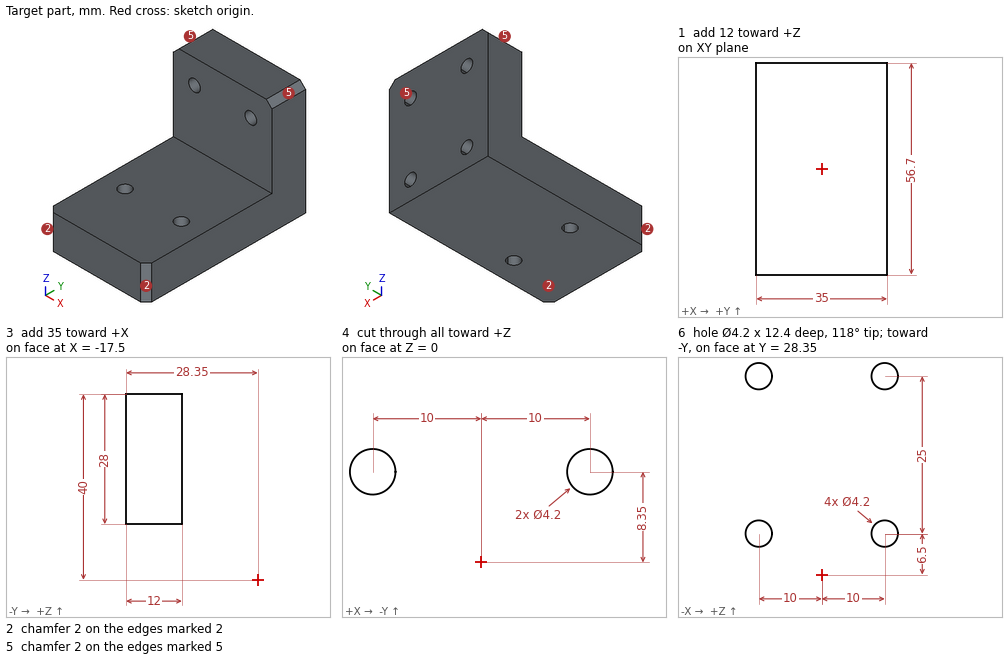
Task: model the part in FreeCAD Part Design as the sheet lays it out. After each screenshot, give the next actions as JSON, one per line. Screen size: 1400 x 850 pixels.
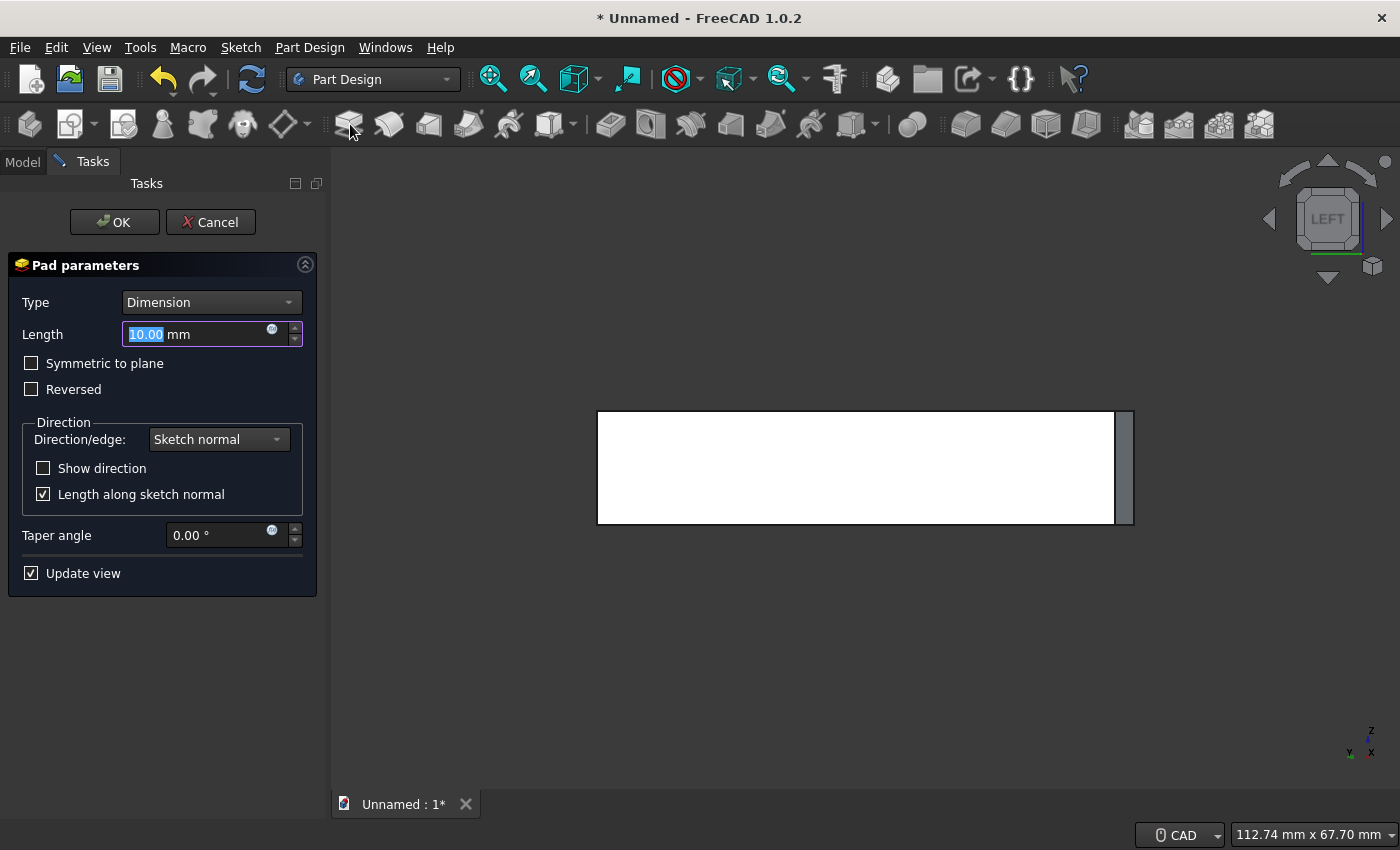
{"action": "type", "text": "35"}
{"action": "key", "text": "Tab"}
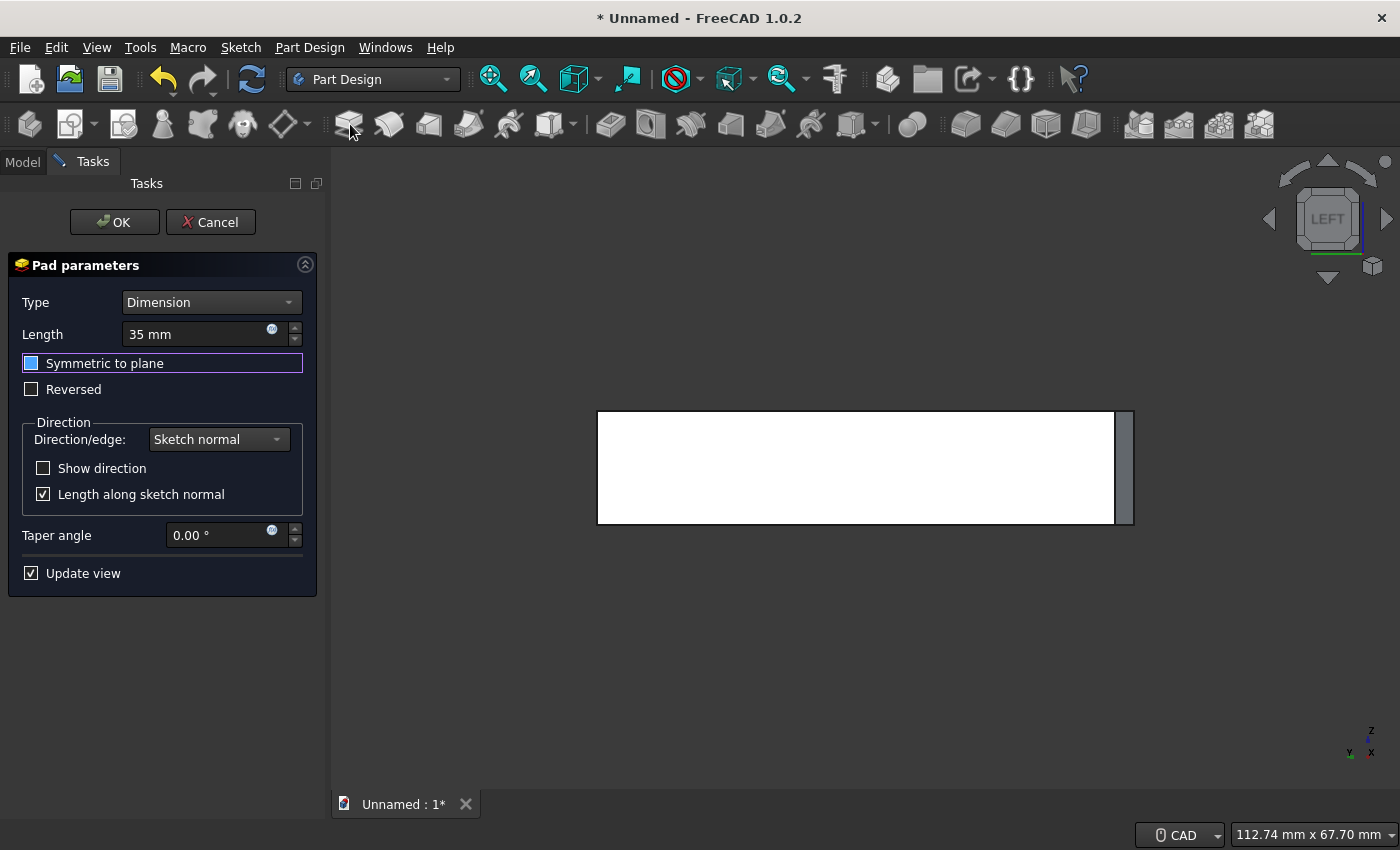
{"action": "left_click", "coordinate": [30, 389]}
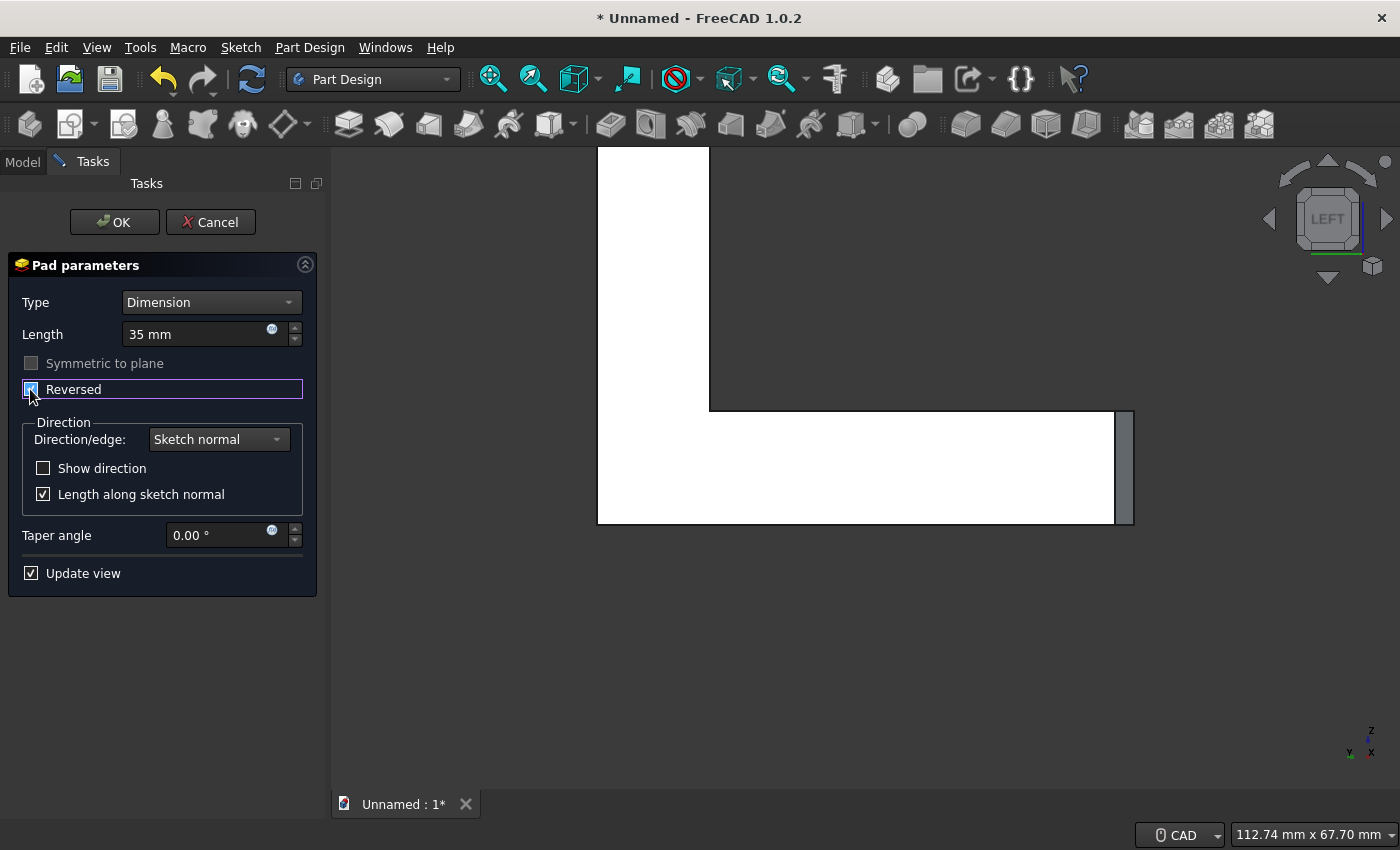
{"action": "left_click", "coordinate": [115, 222]}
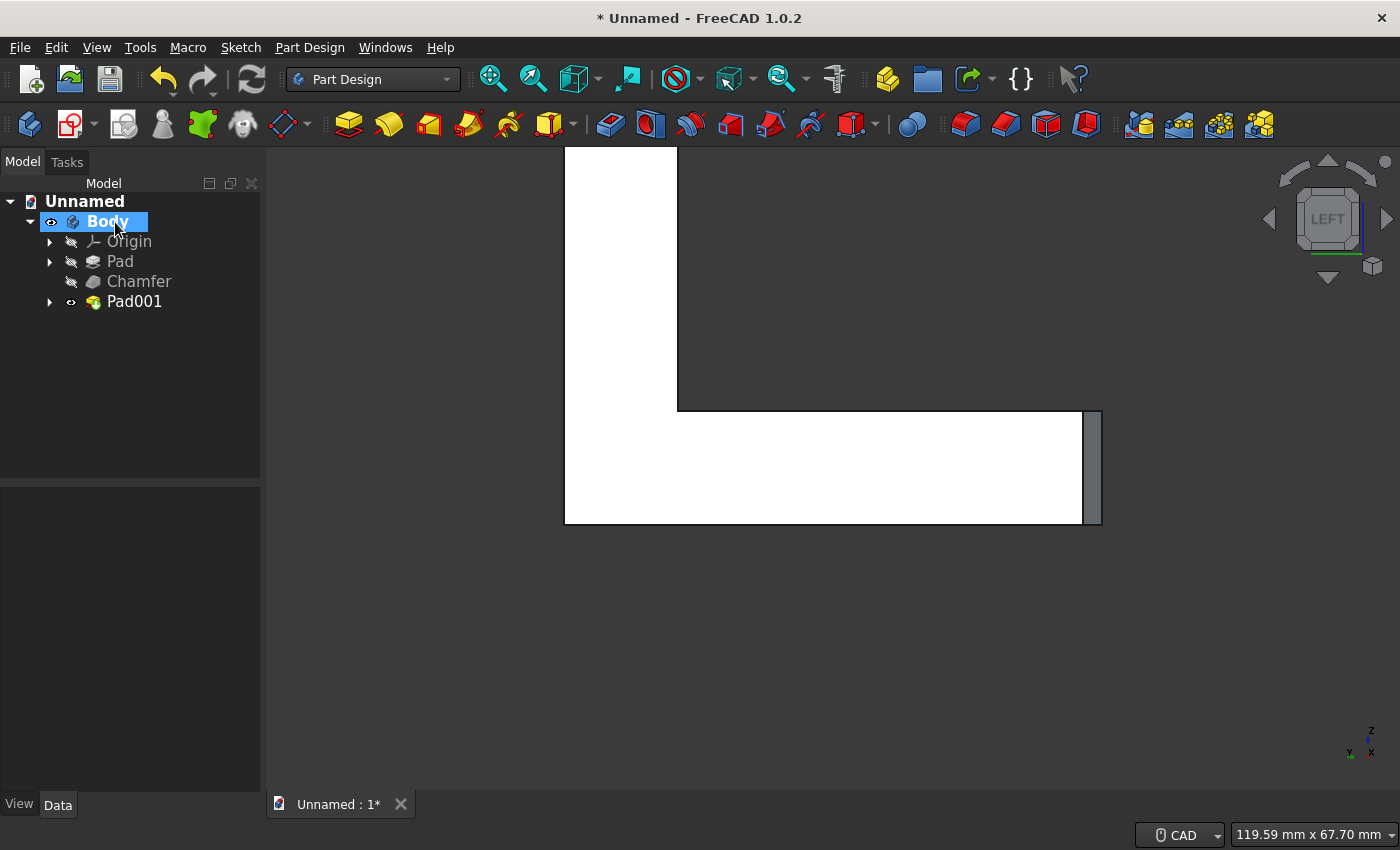
{"action": "left_click", "coordinate": [494, 80]}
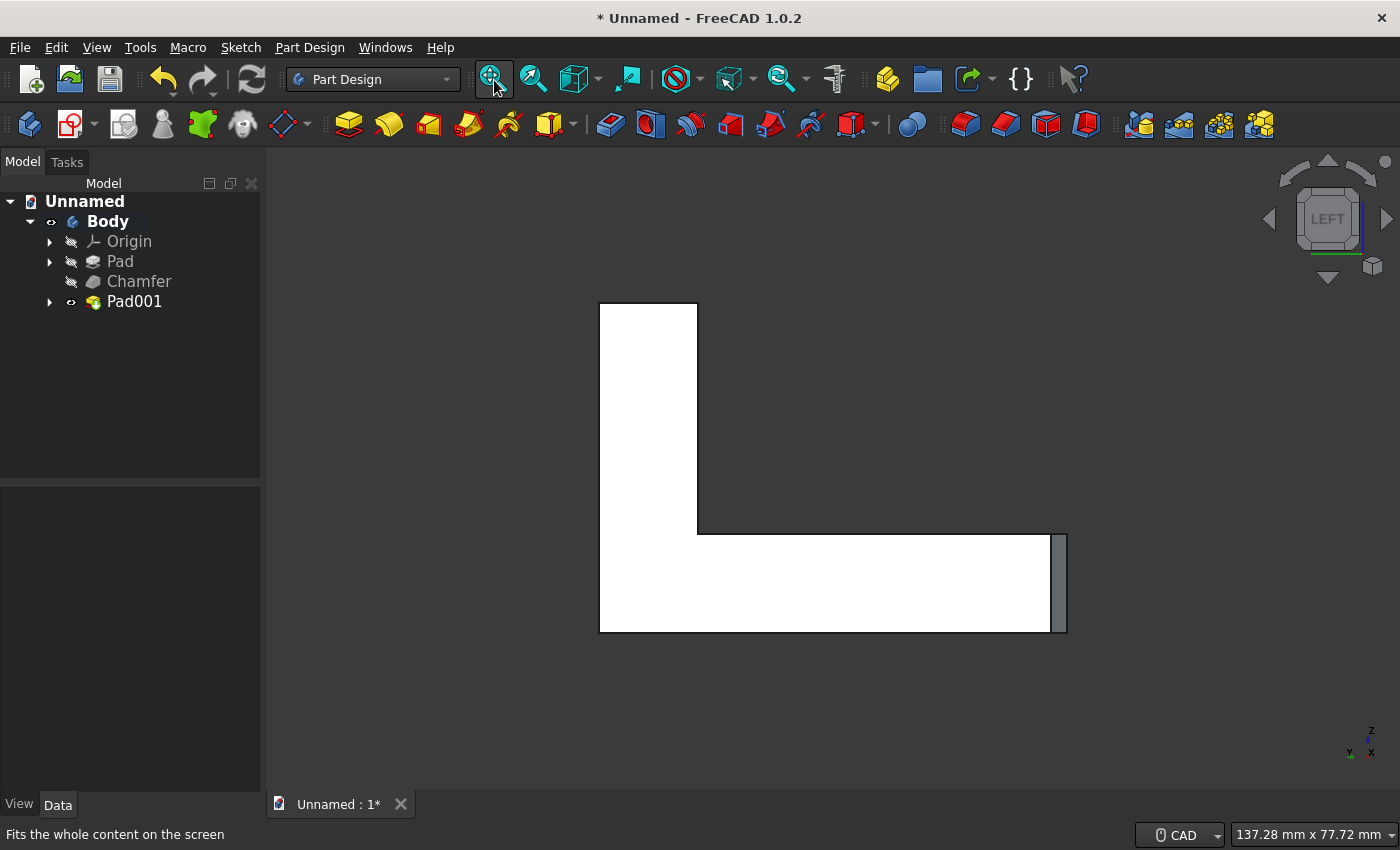
{"action": "key", "text": "5"}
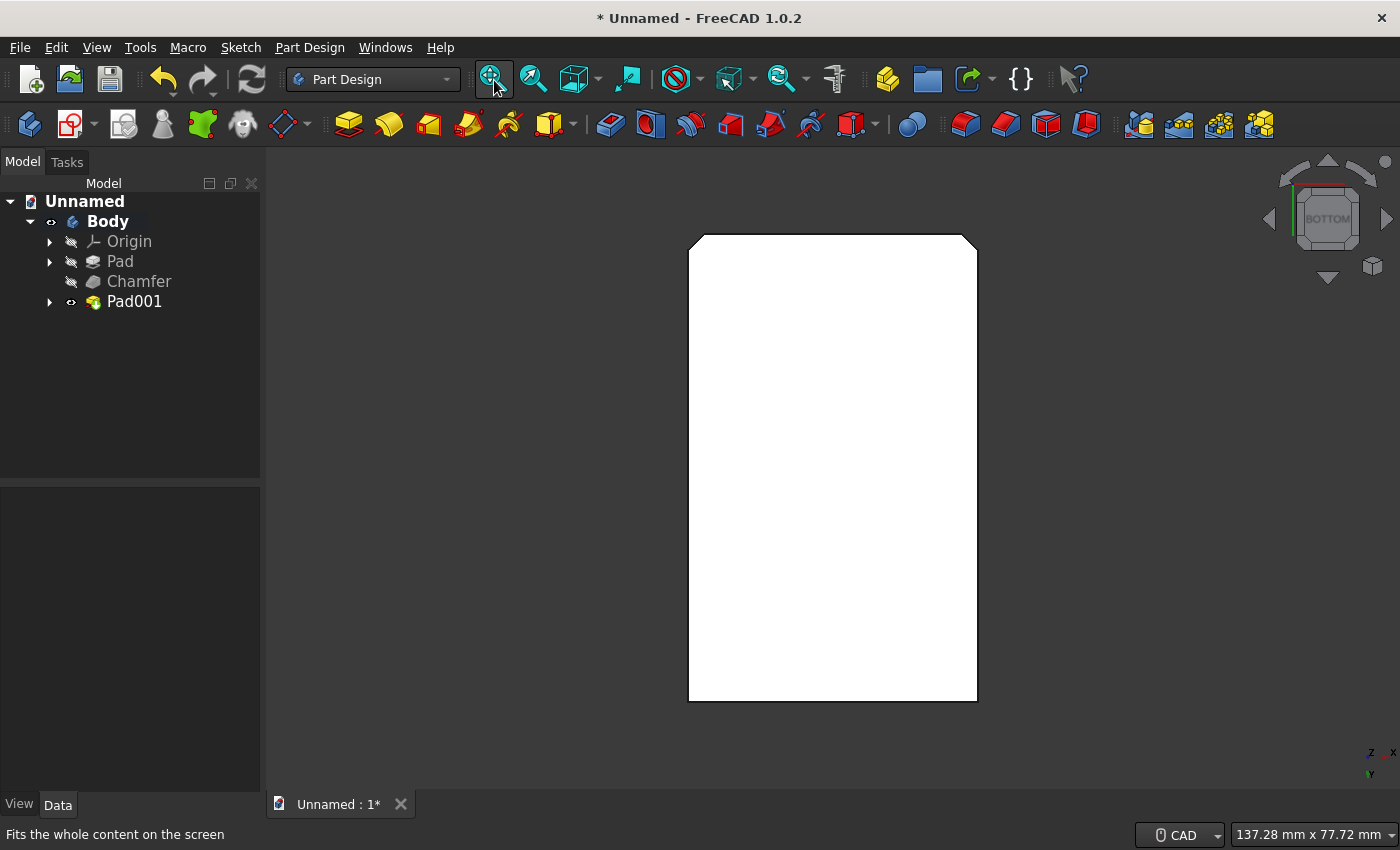
{"action": "left_click", "coordinate": [833, 534]}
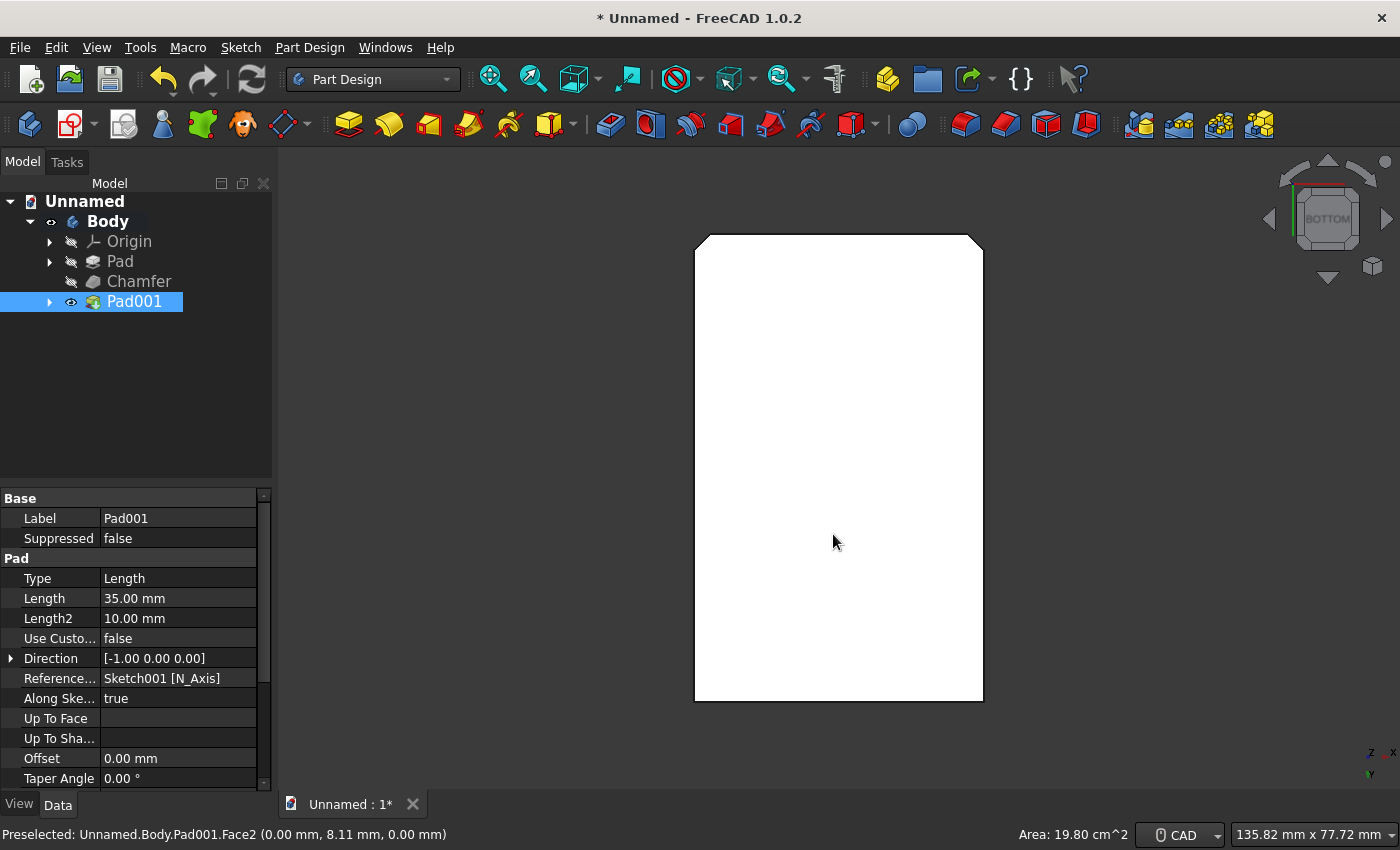
{"action": "left_click", "coordinate": [70, 124]}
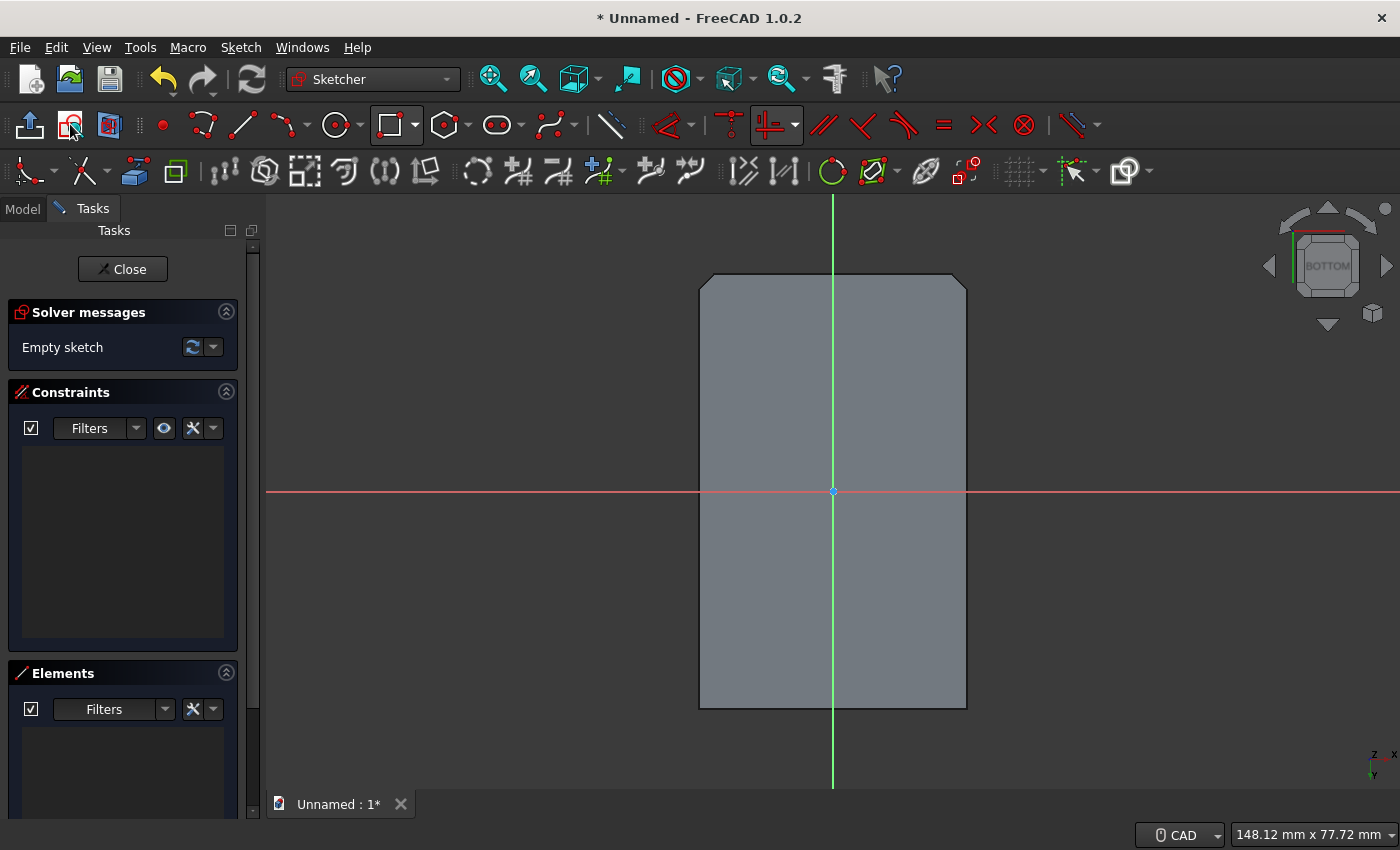
{"action": "scroll", "coordinate": [863, 434], "scroll_direction": "up", "scroll_amount": 6}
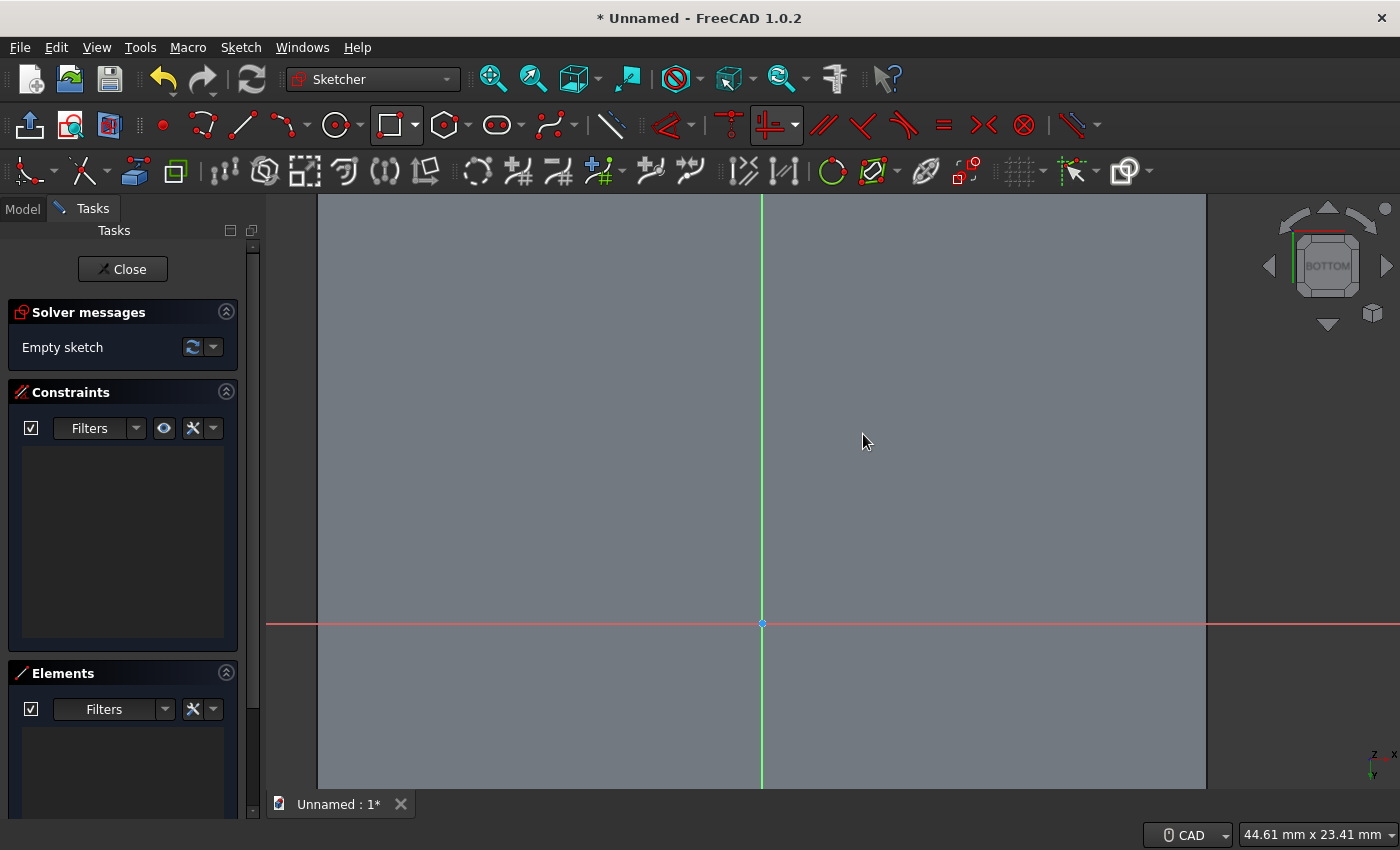
{"action": "left_click", "coordinate": [336, 126]}